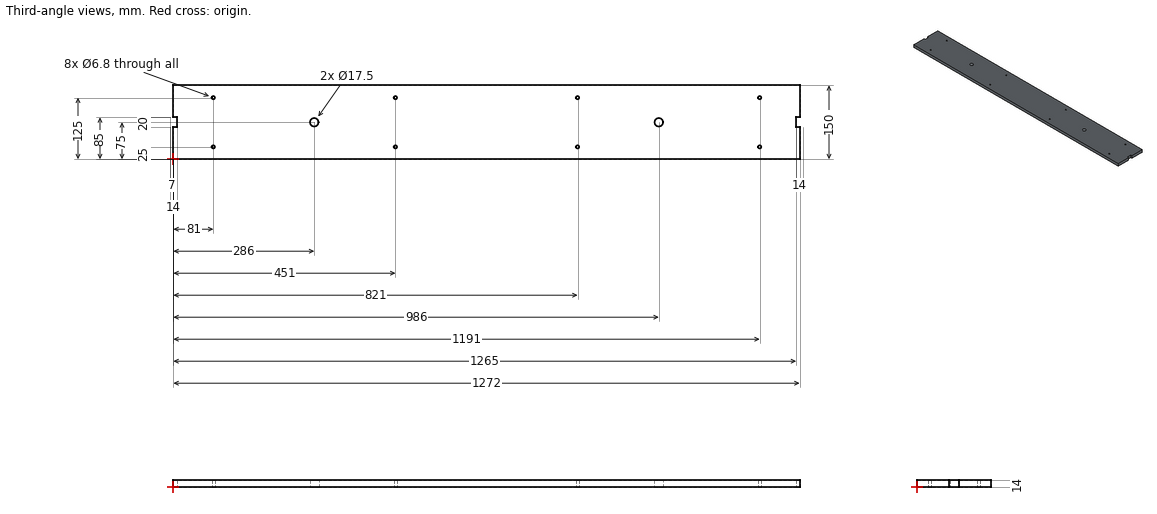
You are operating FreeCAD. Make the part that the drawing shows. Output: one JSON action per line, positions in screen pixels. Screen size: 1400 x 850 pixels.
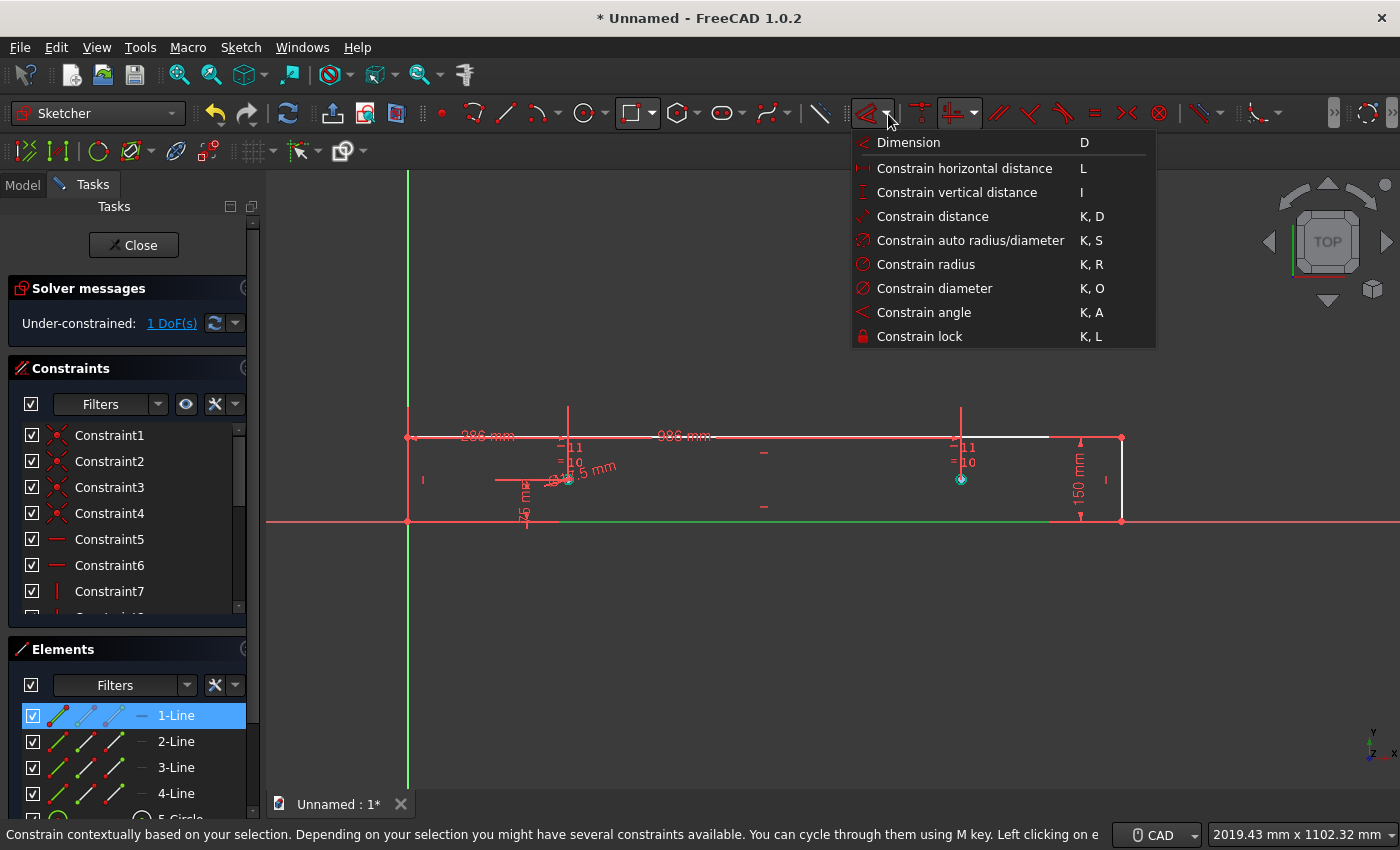
{"action": "left_click", "coordinate": [1004, 168]}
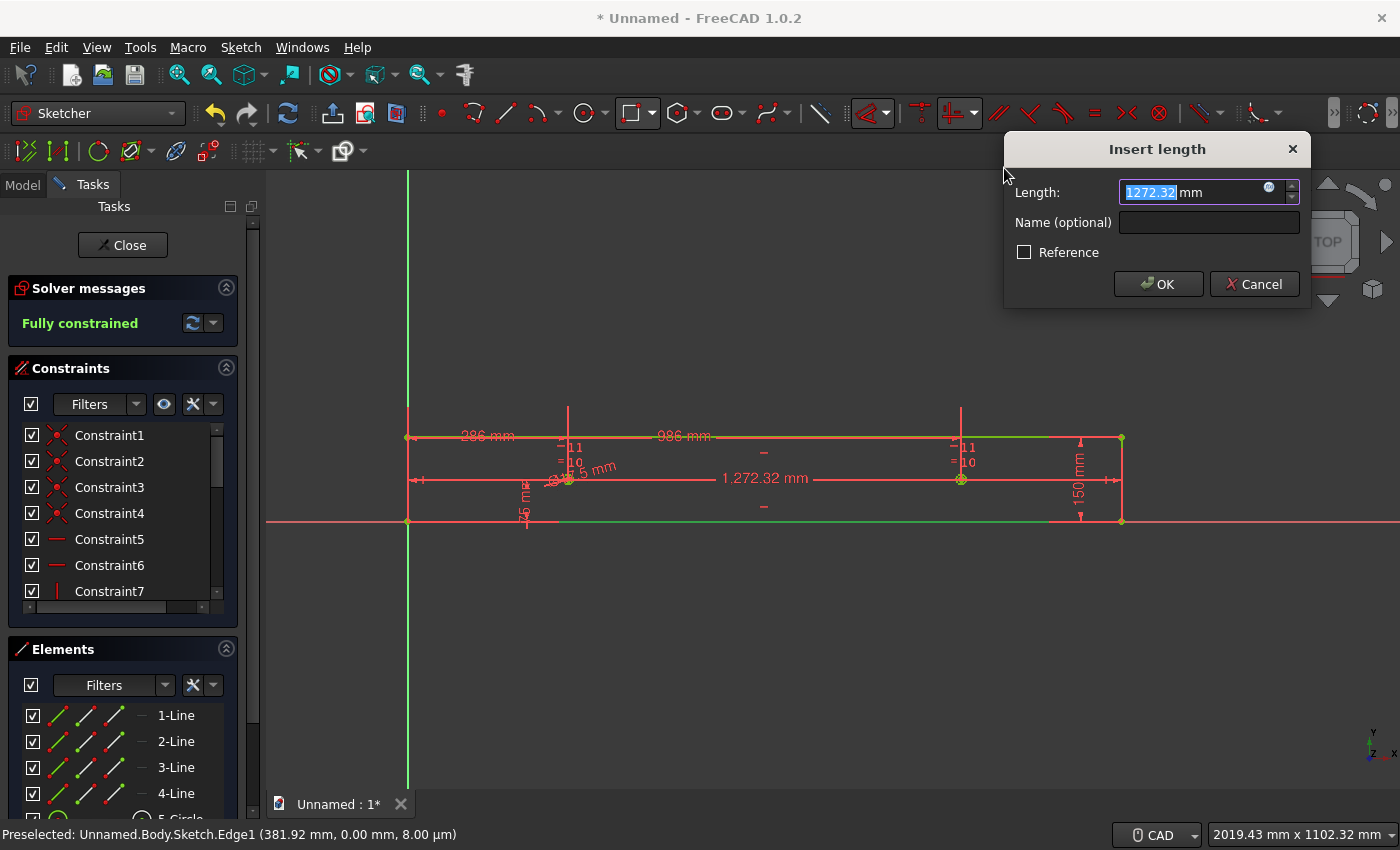
{"action": "type", "text": "1272"}
{"action": "key", "text": "Return"}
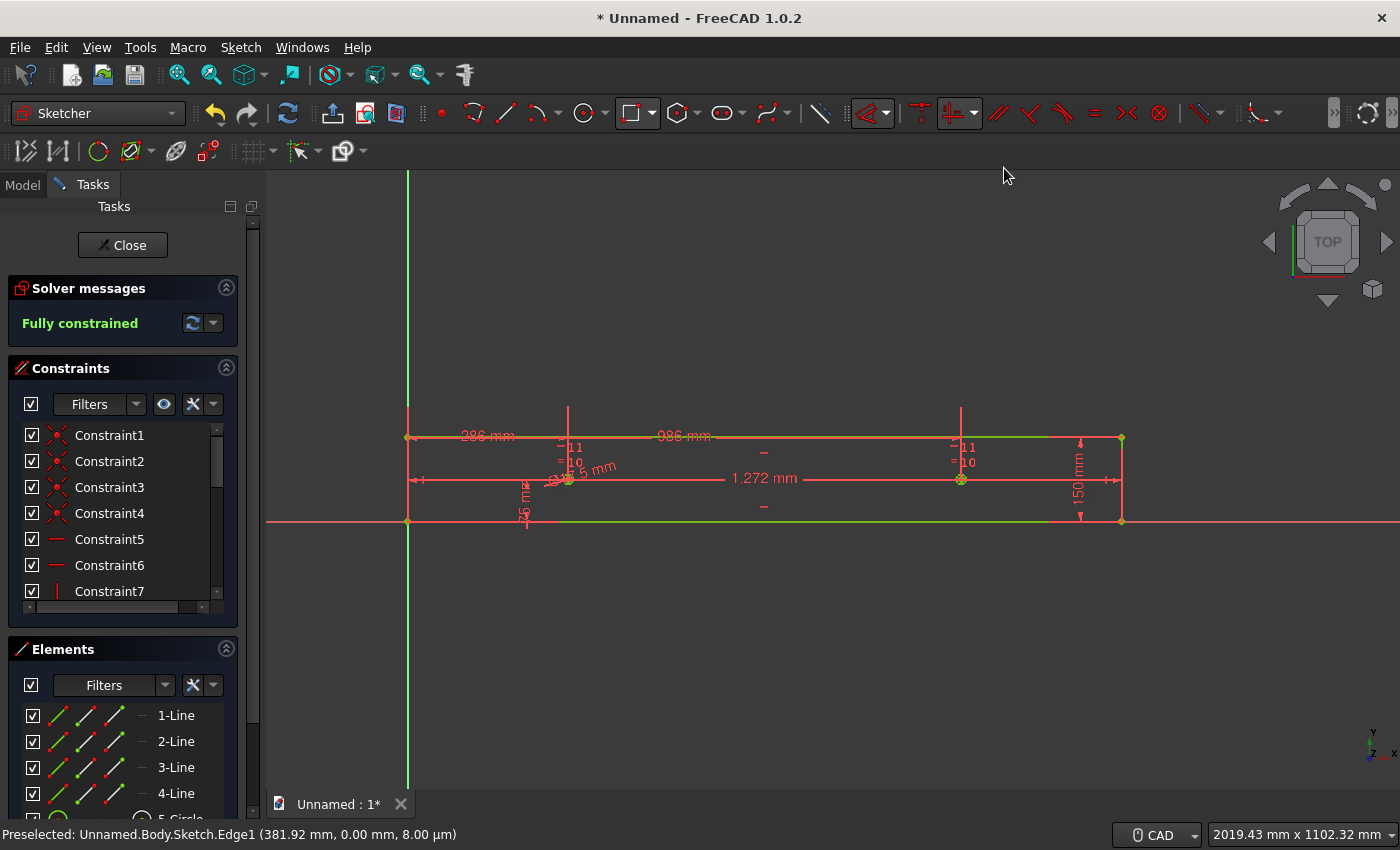
{"action": "left_click", "coordinate": [123, 245]}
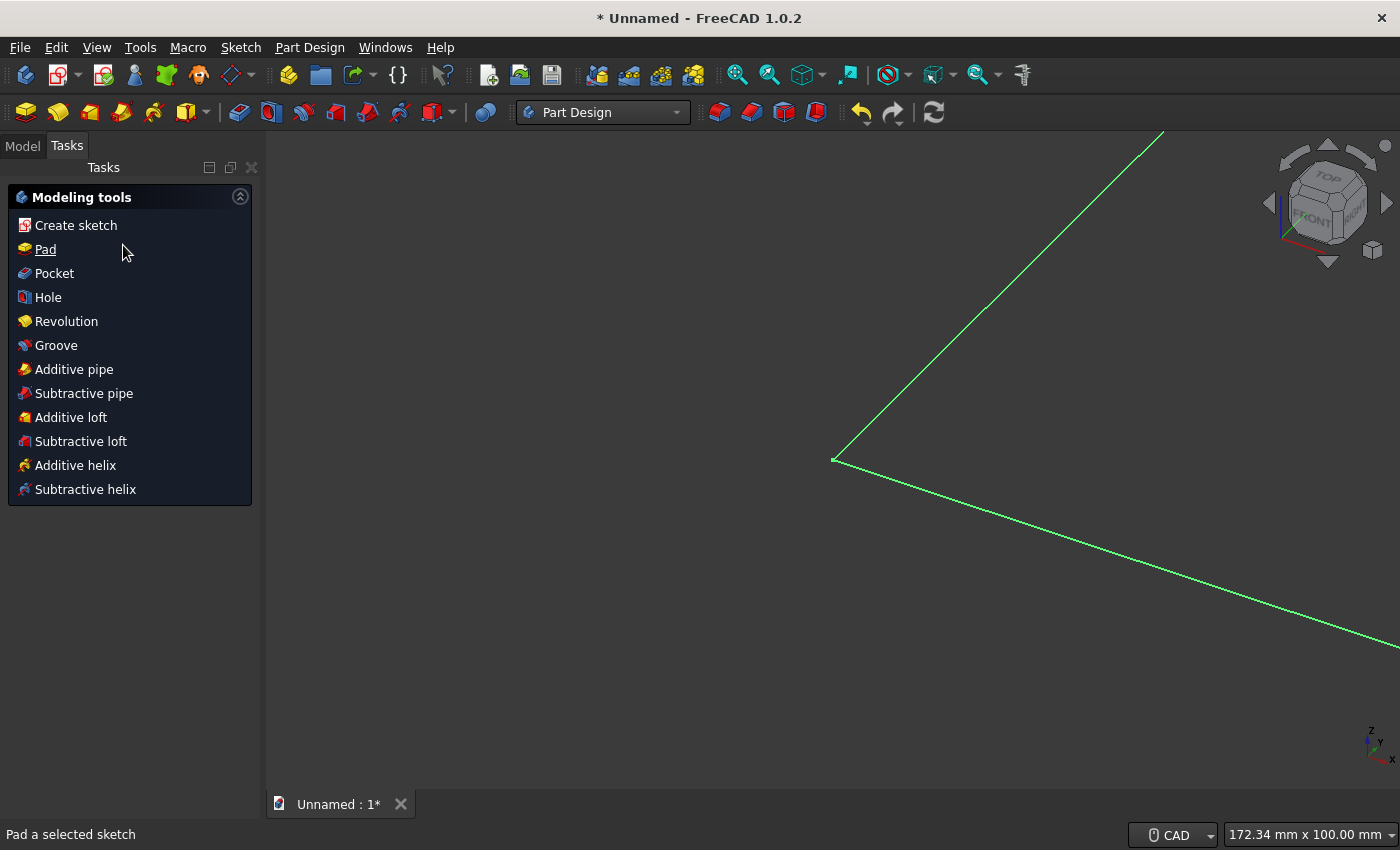
{"action": "left_click", "coordinate": [26, 112]}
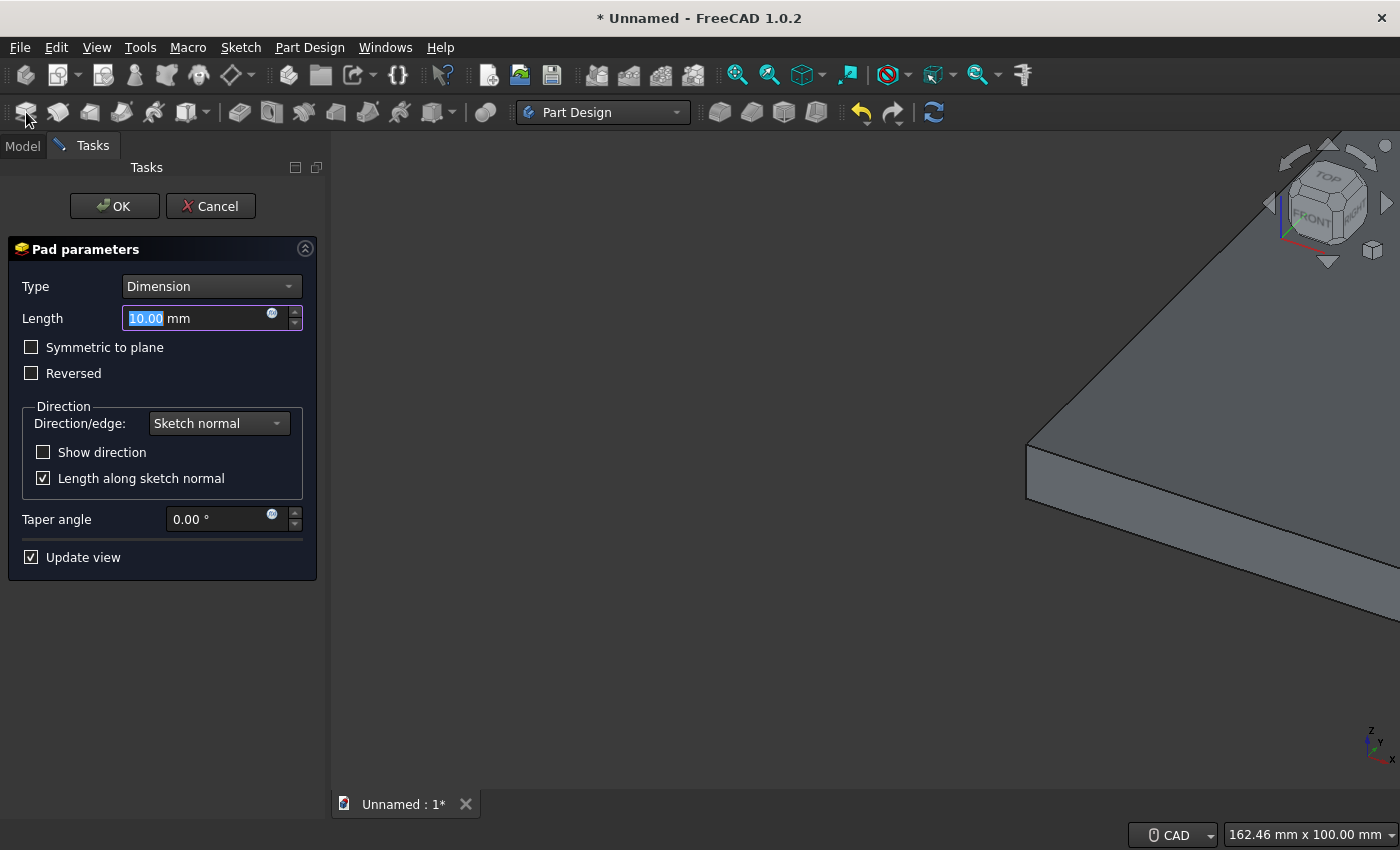
{"action": "type", "text": "14"}
{"action": "key", "text": "Tab"}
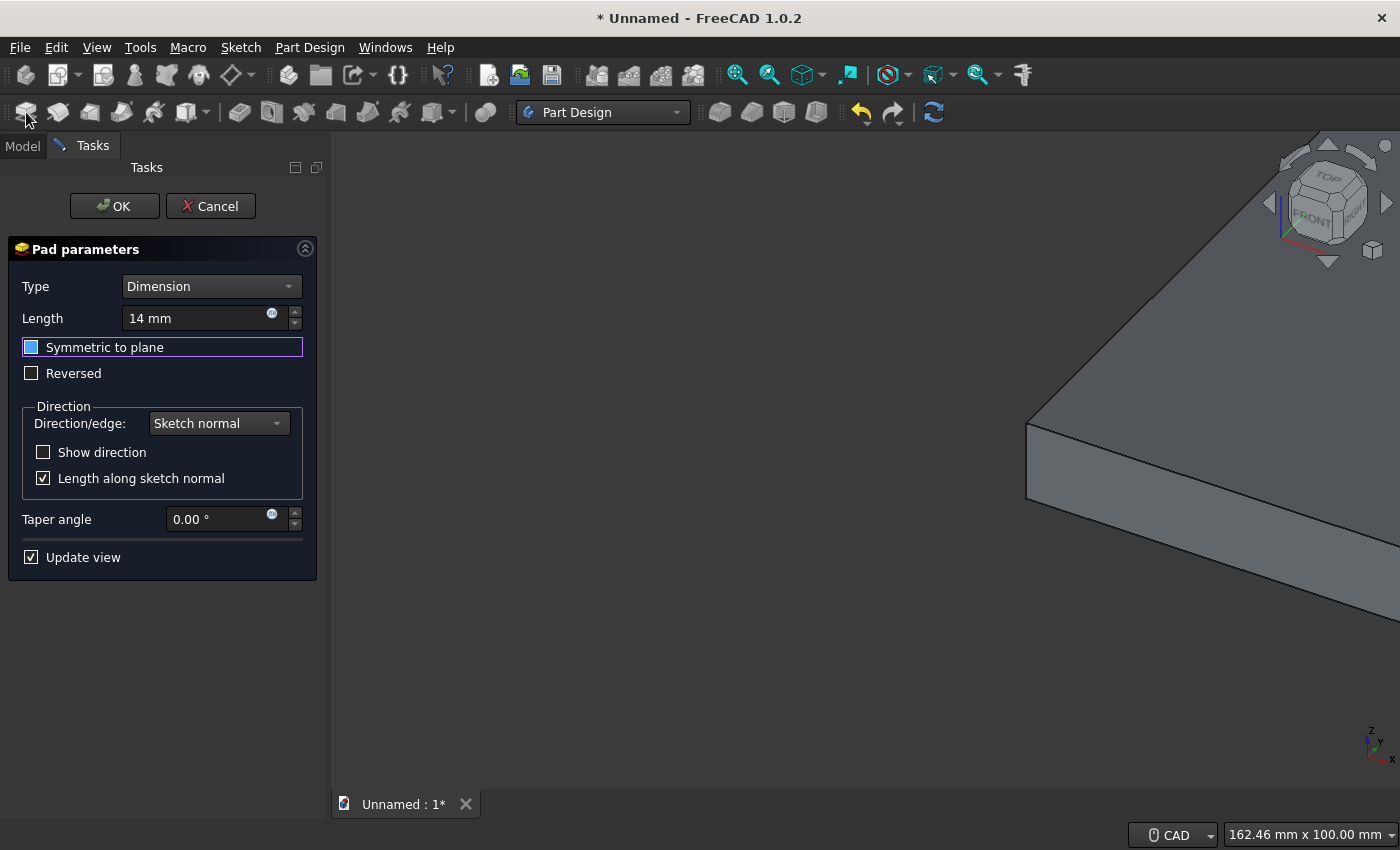
{"action": "left_click", "coordinate": [115, 206]}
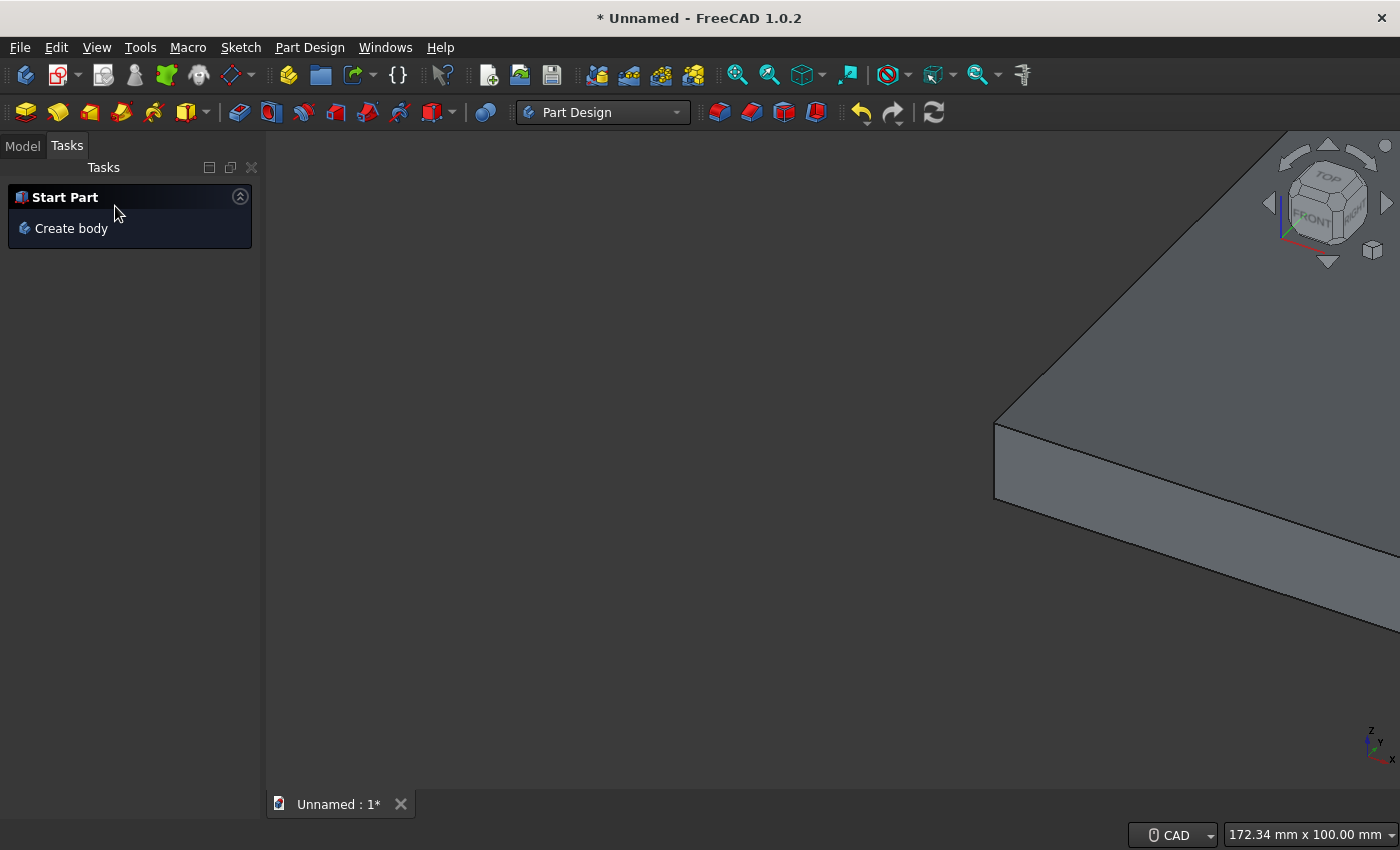
{"action": "left_click", "coordinate": [738, 76]}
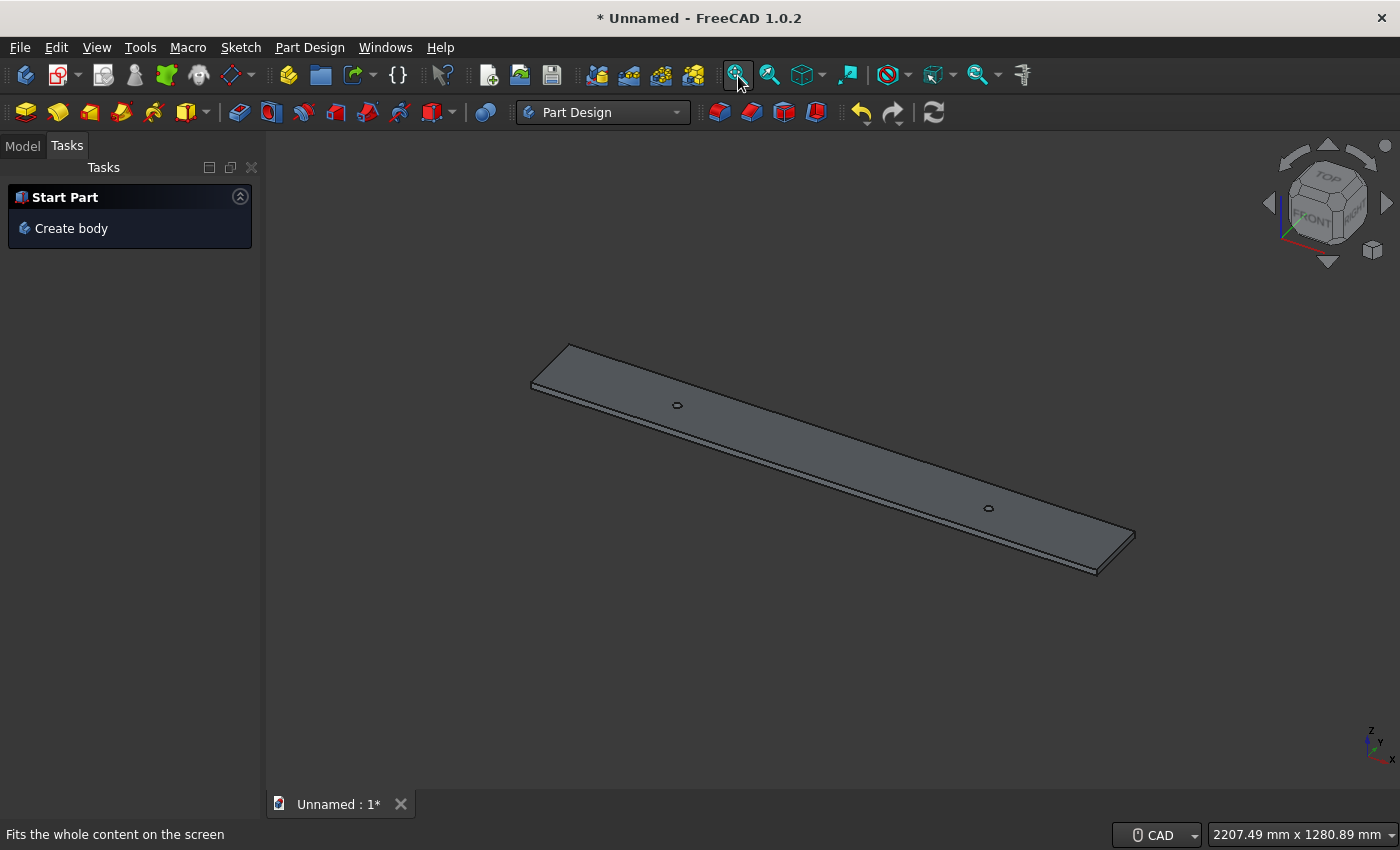
{"action": "left_click", "coordinate": [1076, 536]}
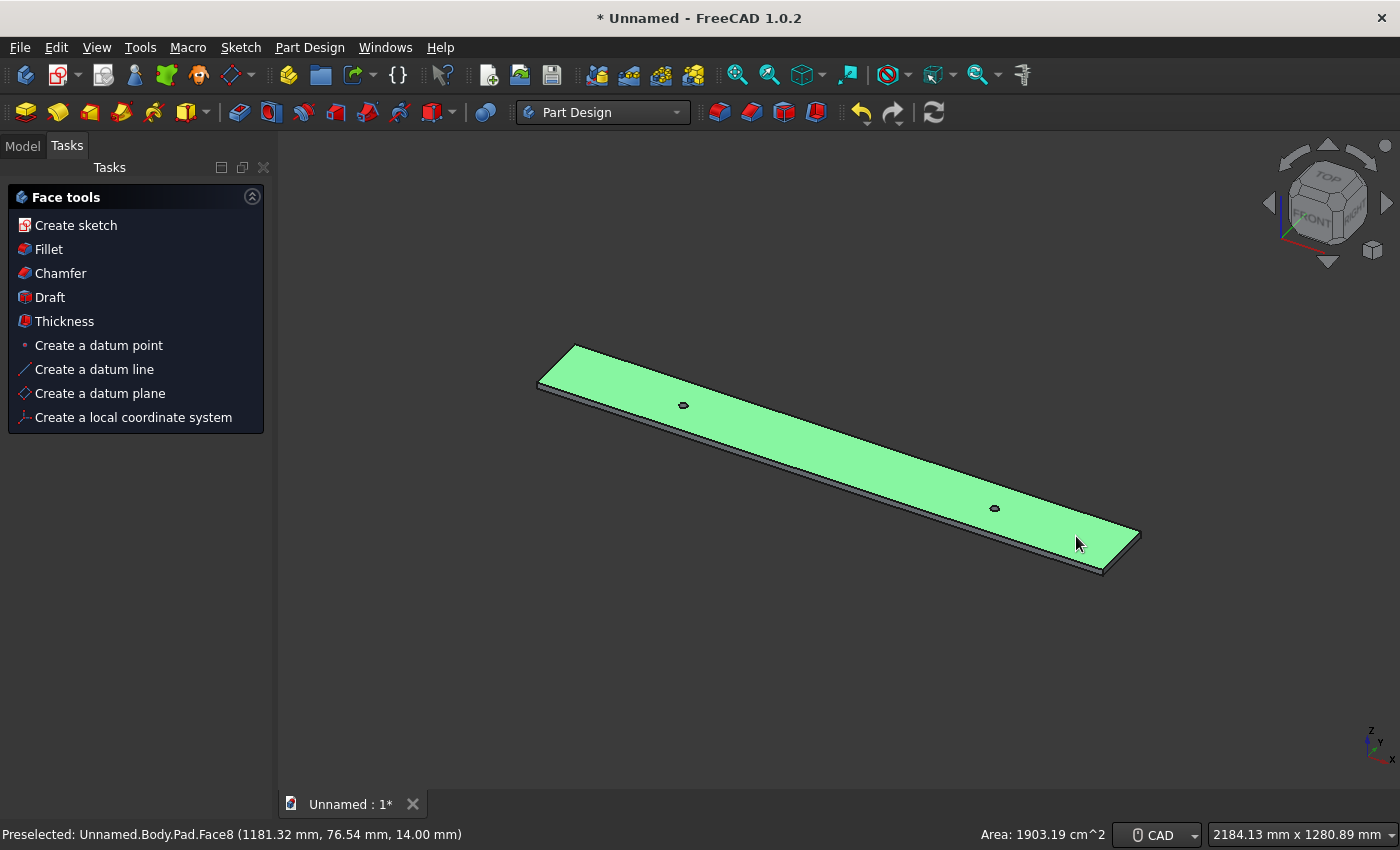
{"action": "left_click", "coordinate": [58, 76]}